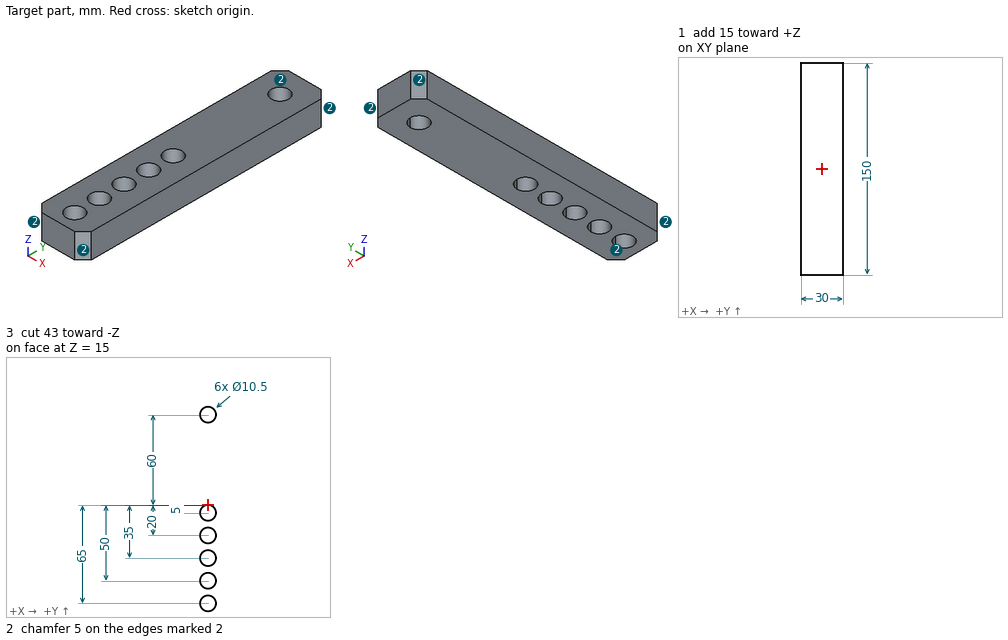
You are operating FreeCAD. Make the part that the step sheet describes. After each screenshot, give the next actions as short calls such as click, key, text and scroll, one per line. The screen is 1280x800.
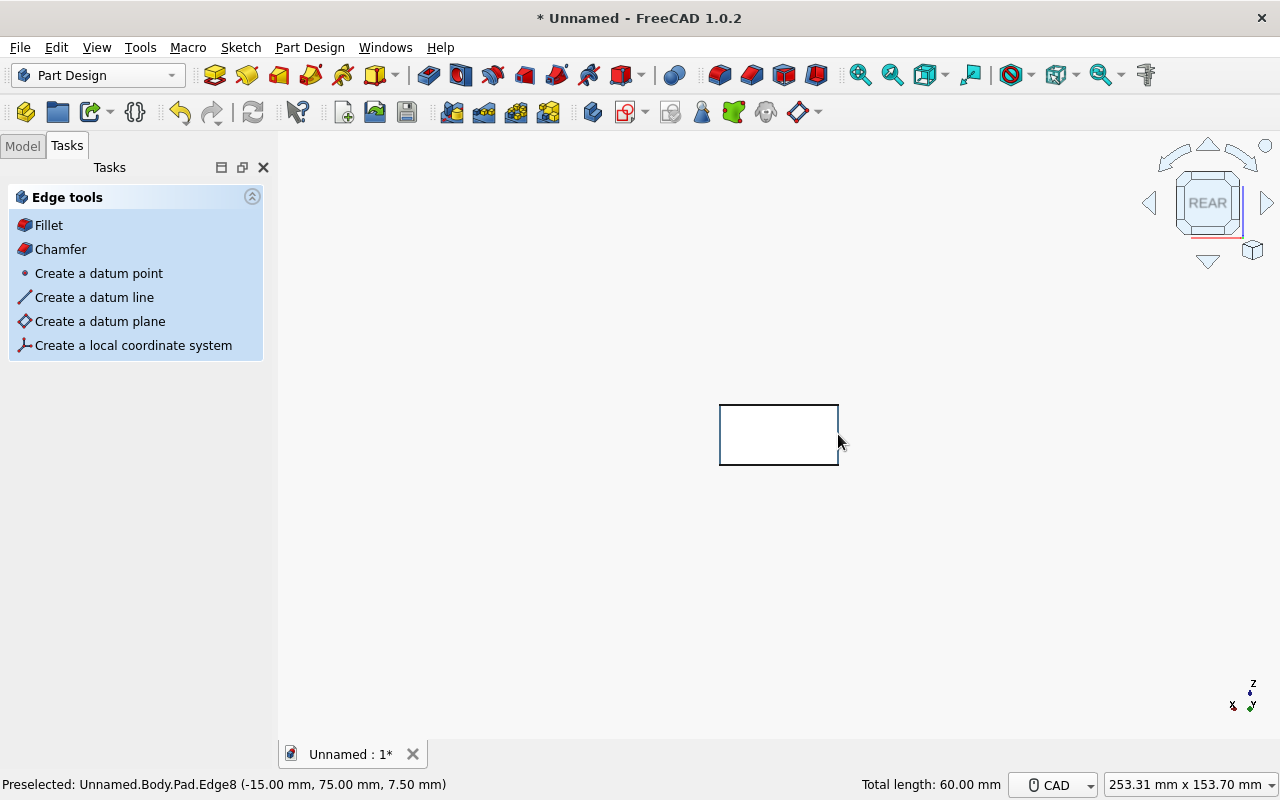
click(752, 76)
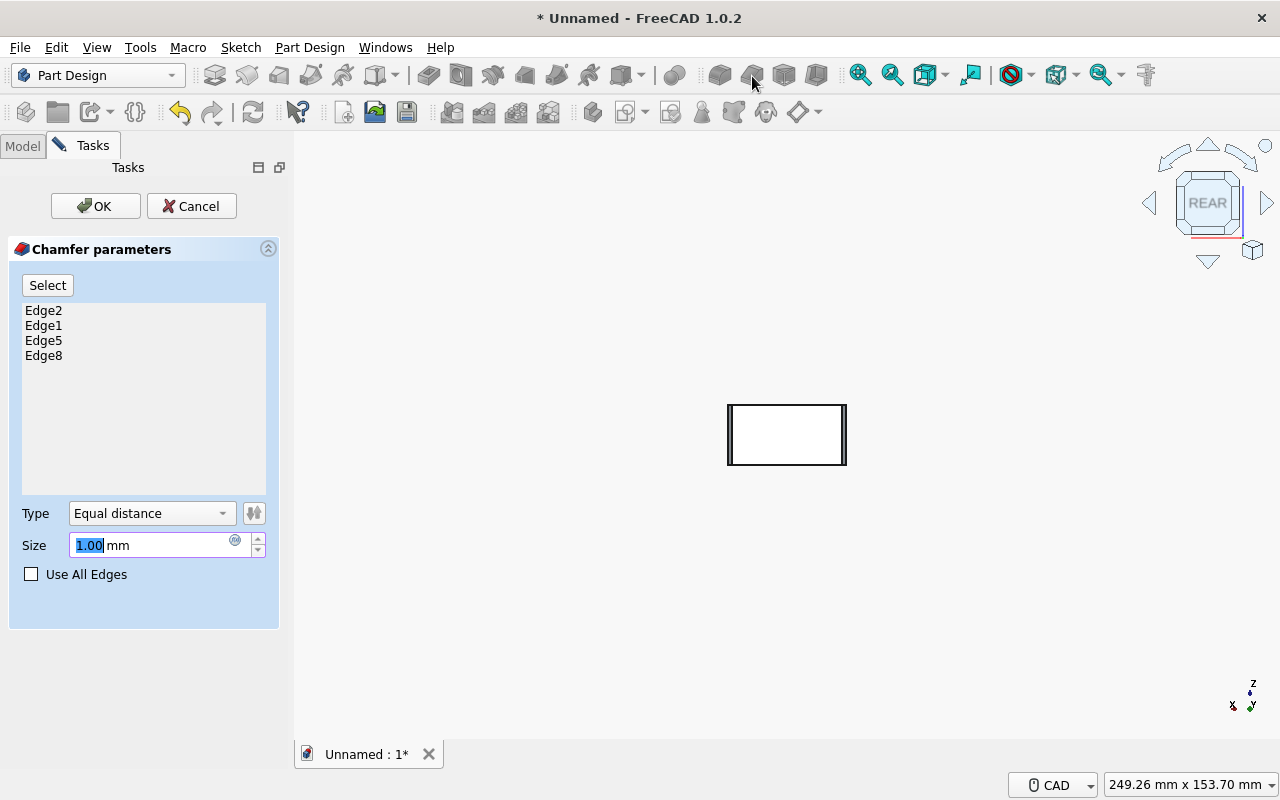
text(5)
key(Tab)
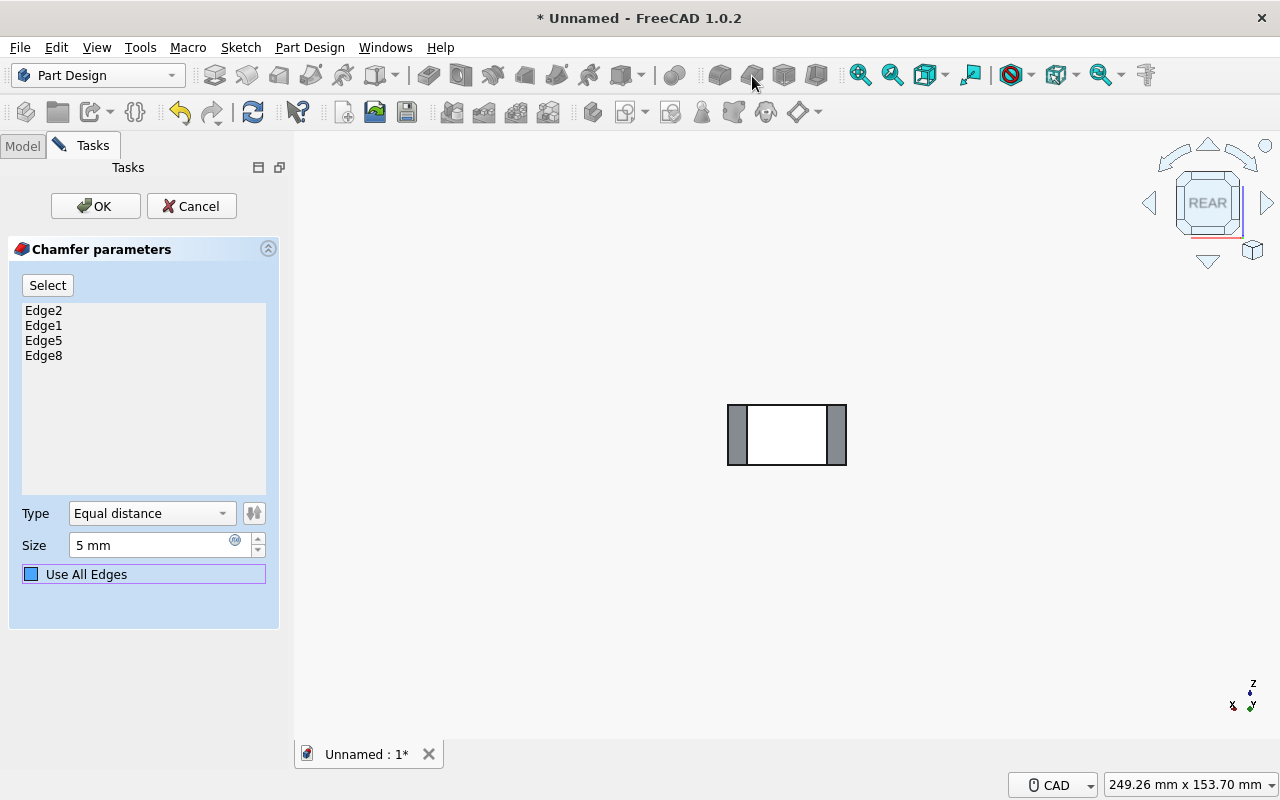
click(96, 206)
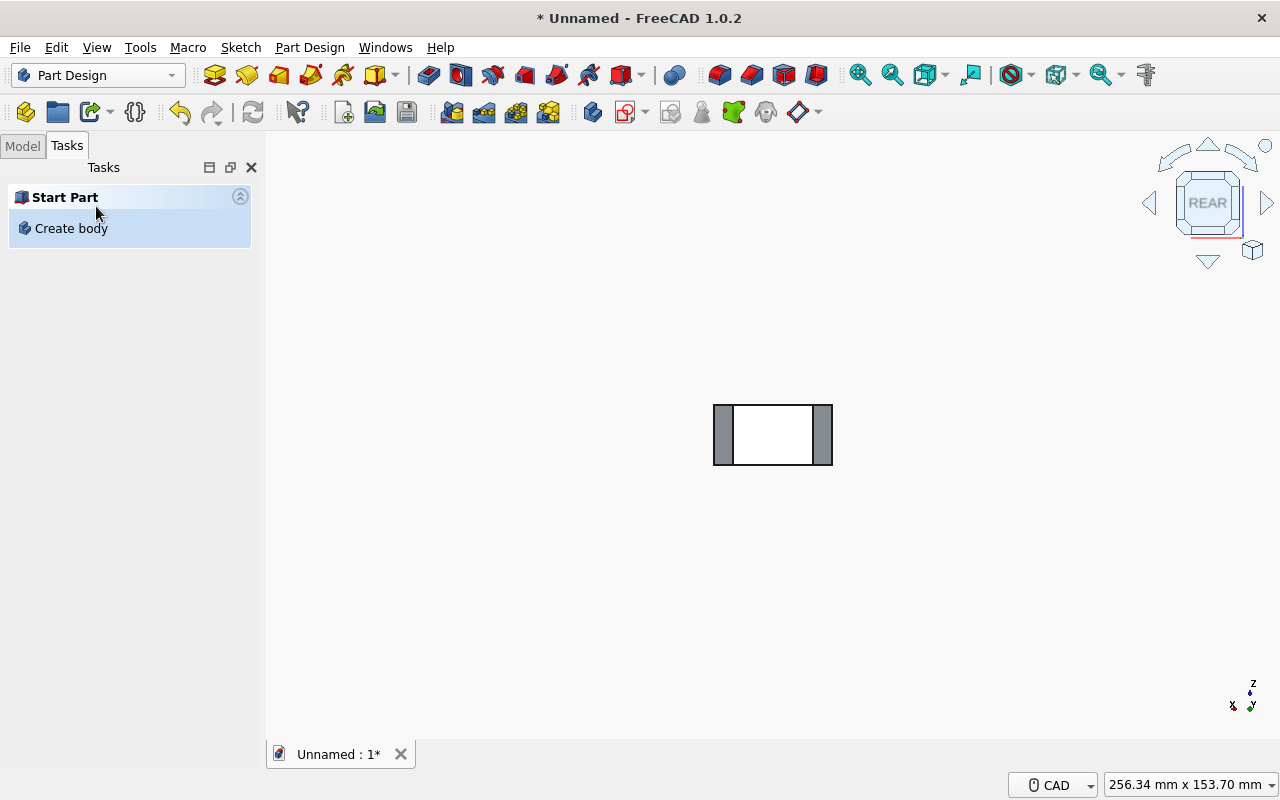
click(862, 76)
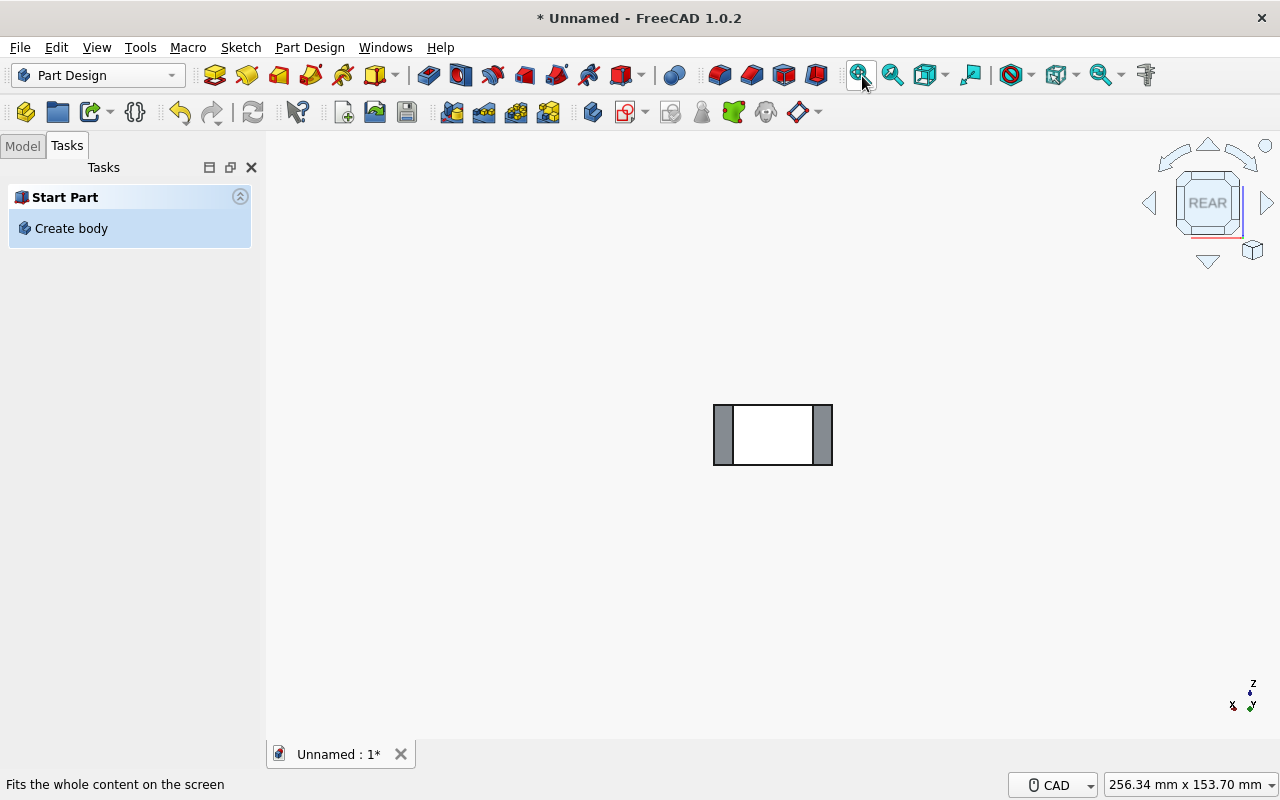
key(0)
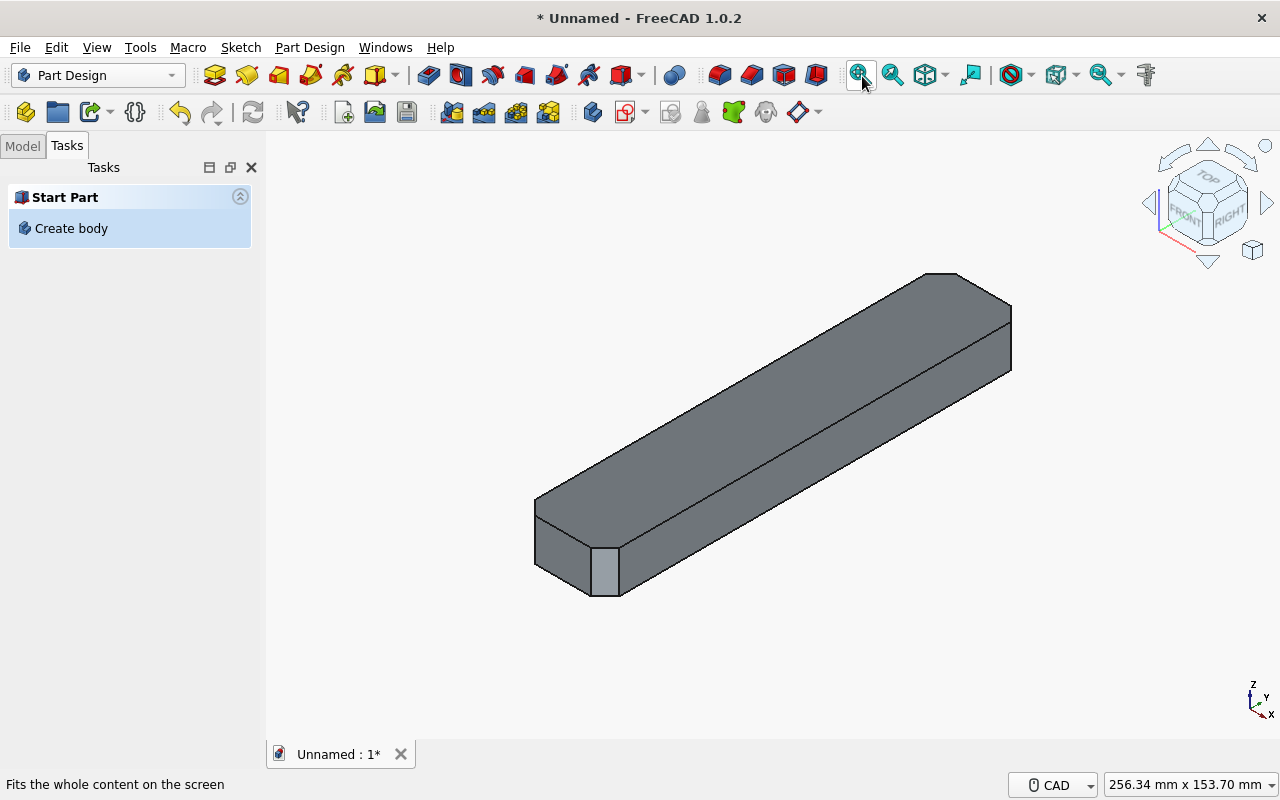
click(893, 341)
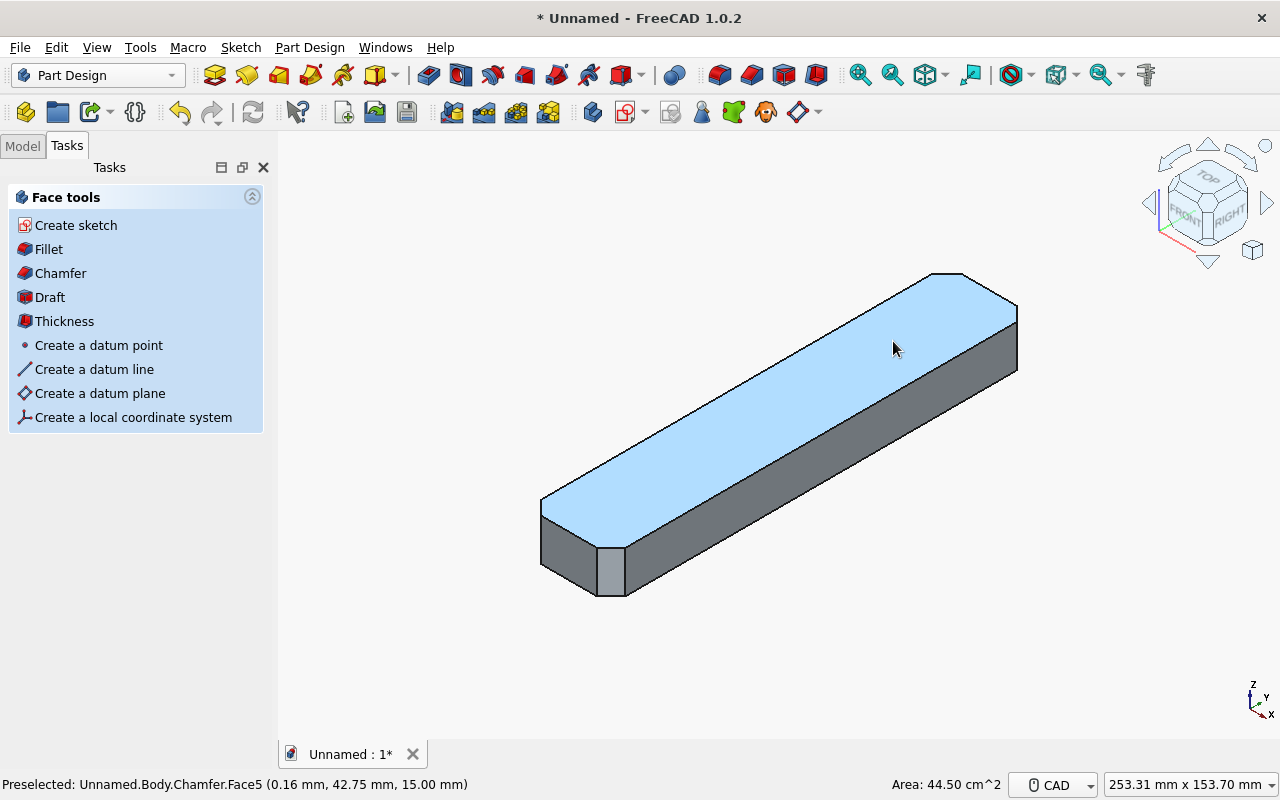
click(626, 112)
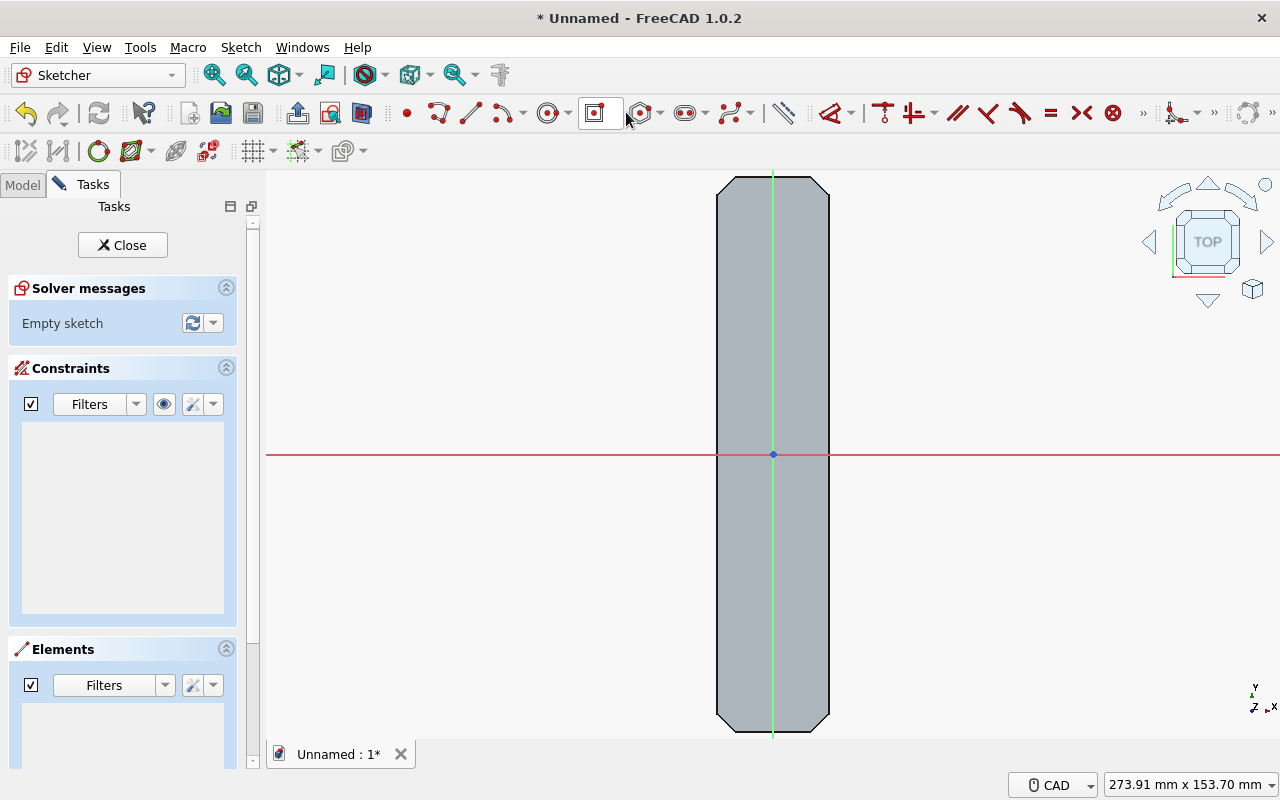
scroll(565, 436, down, 2)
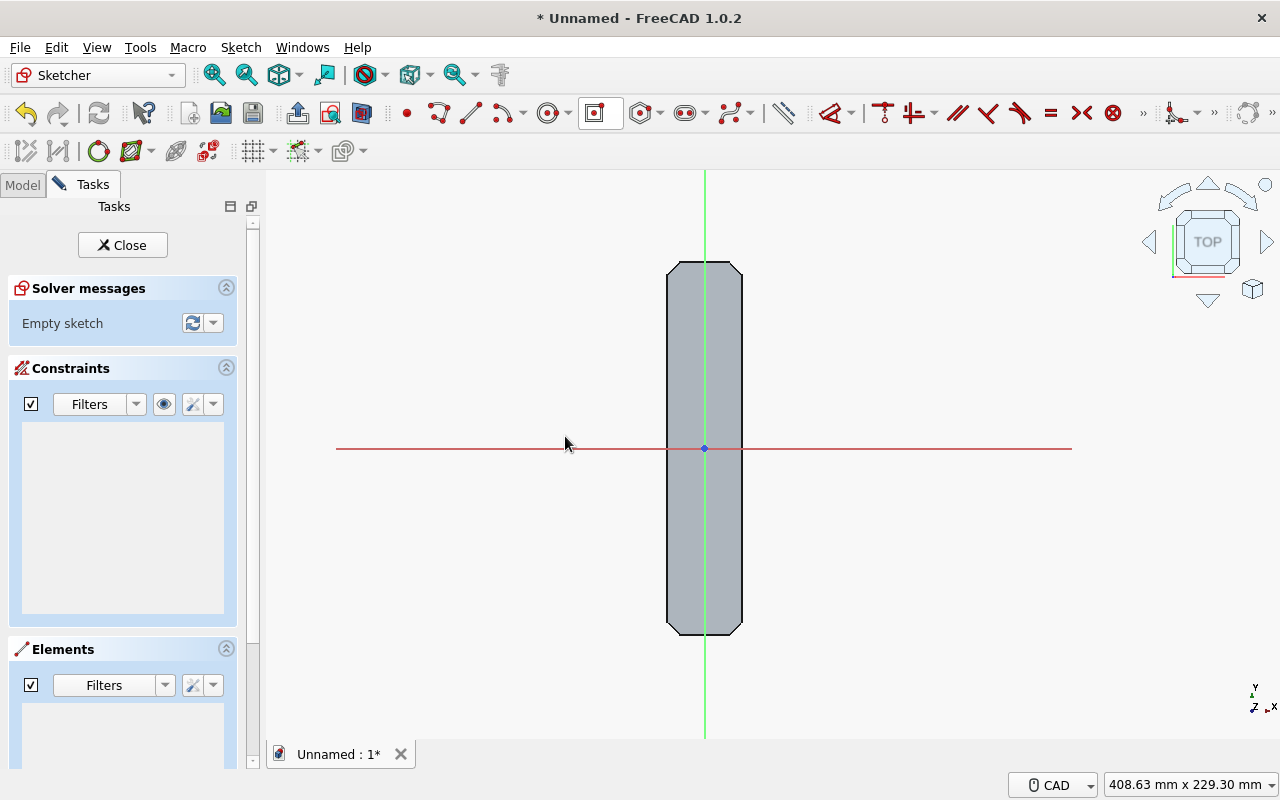
click(548, 114)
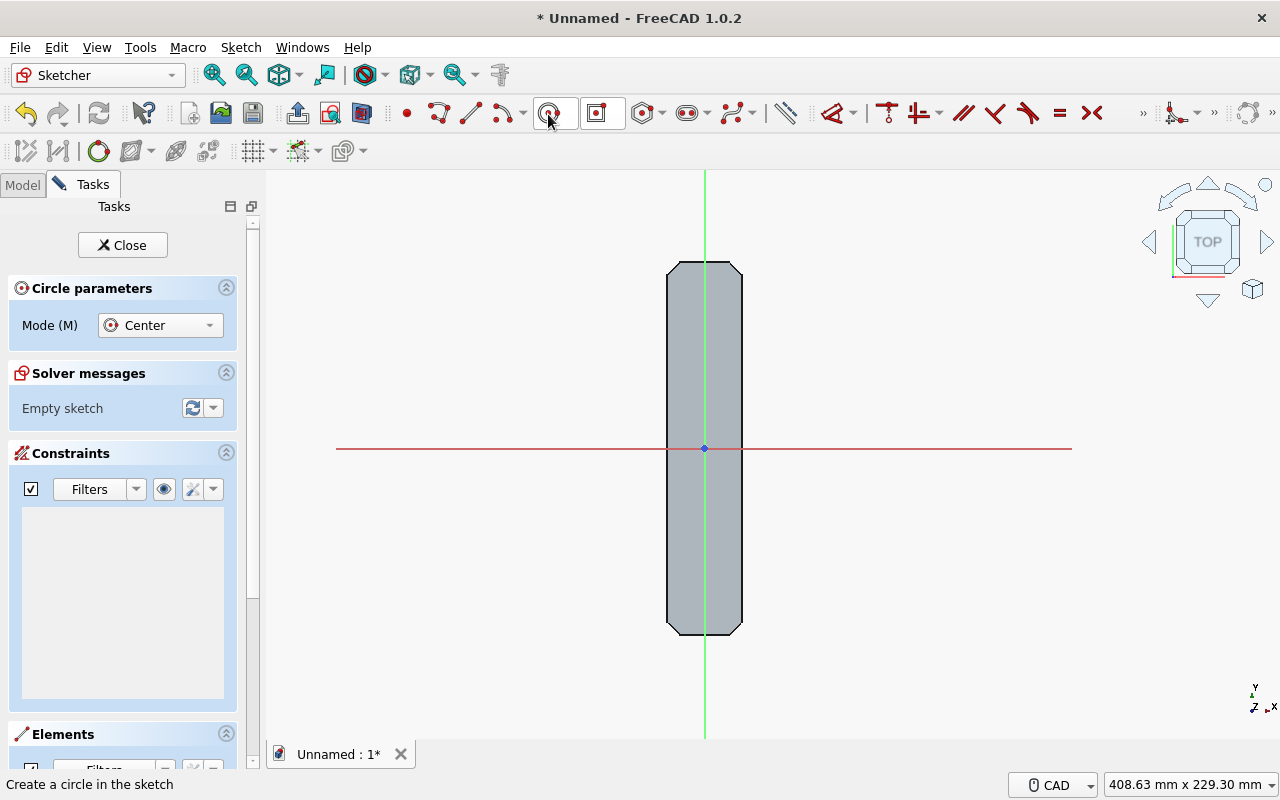
scroll(705, 300, up, 3)